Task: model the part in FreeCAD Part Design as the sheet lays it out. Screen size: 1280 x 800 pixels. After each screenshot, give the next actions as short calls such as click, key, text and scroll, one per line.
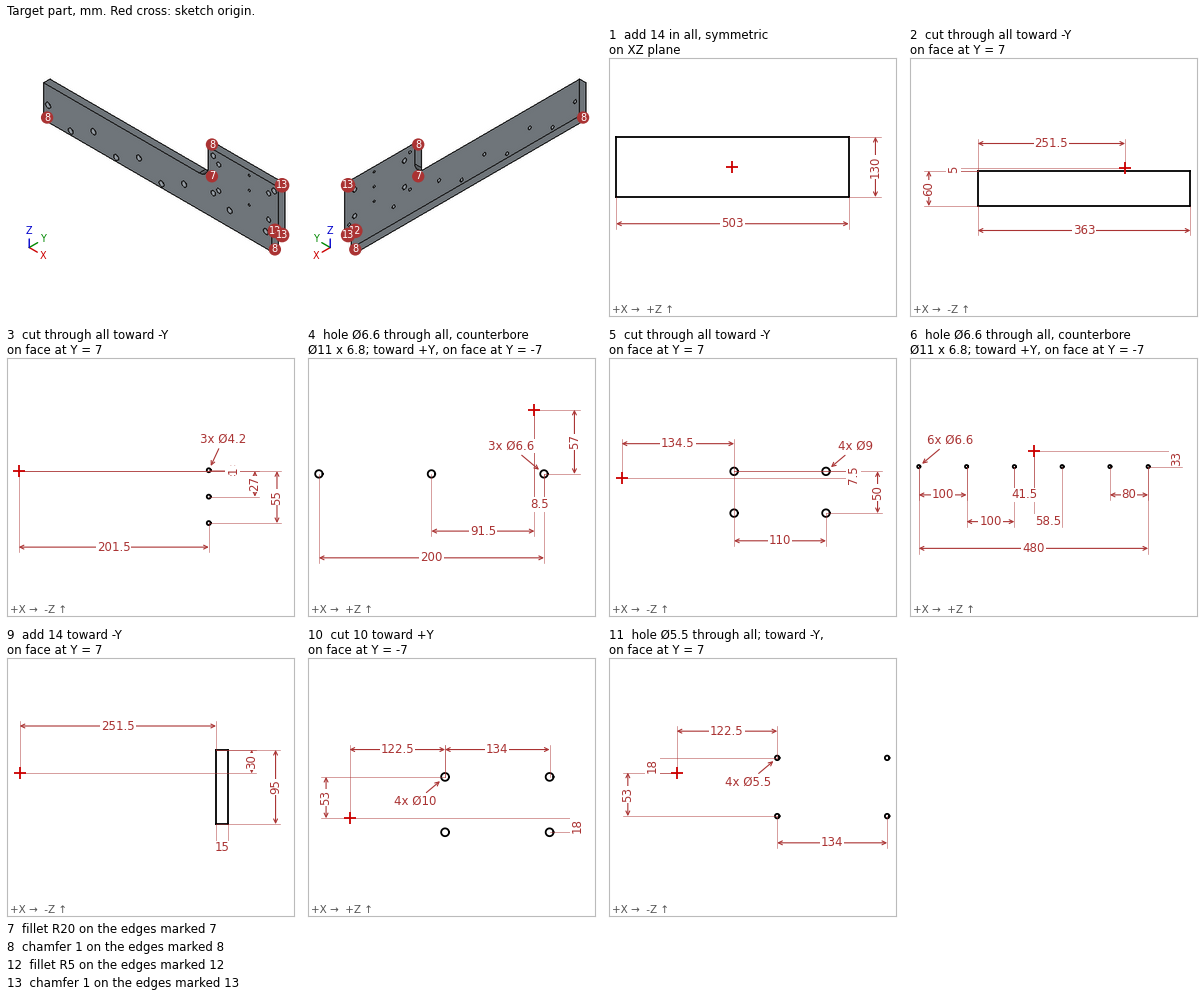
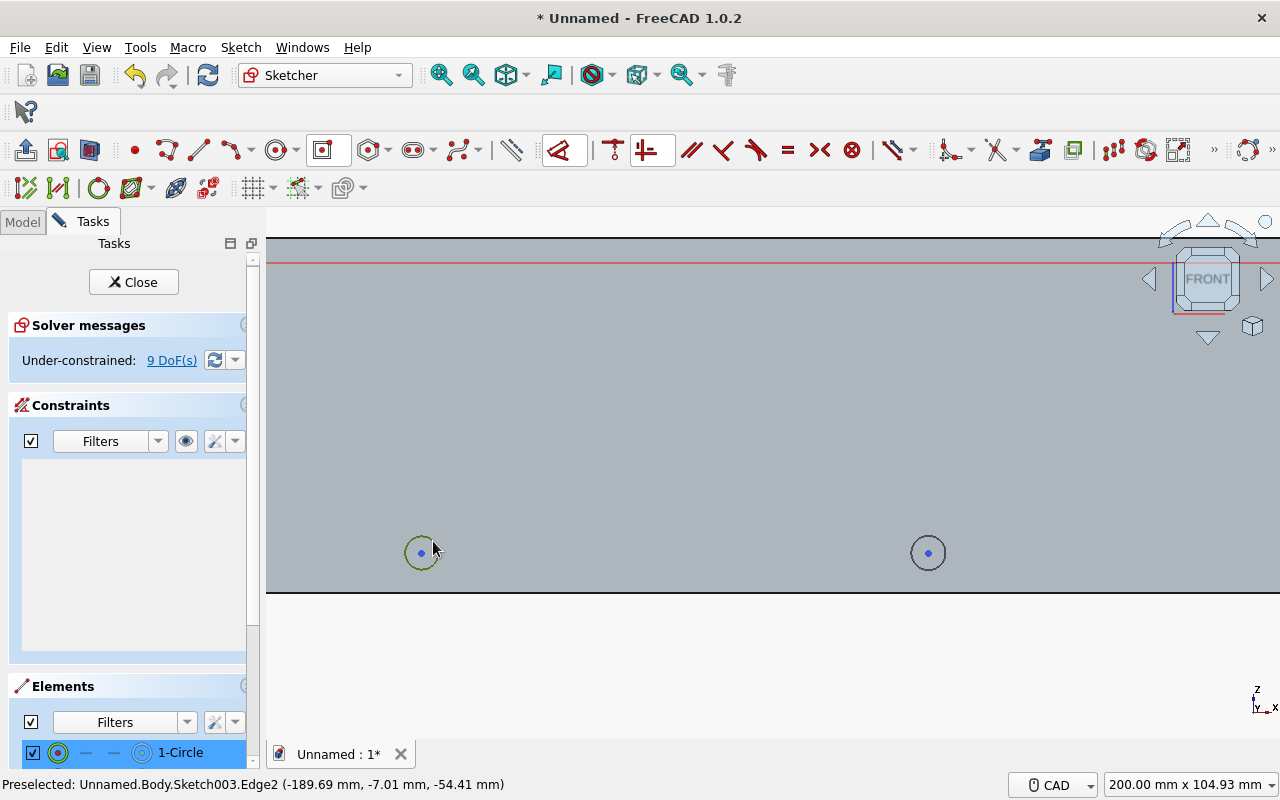
click(940, 541)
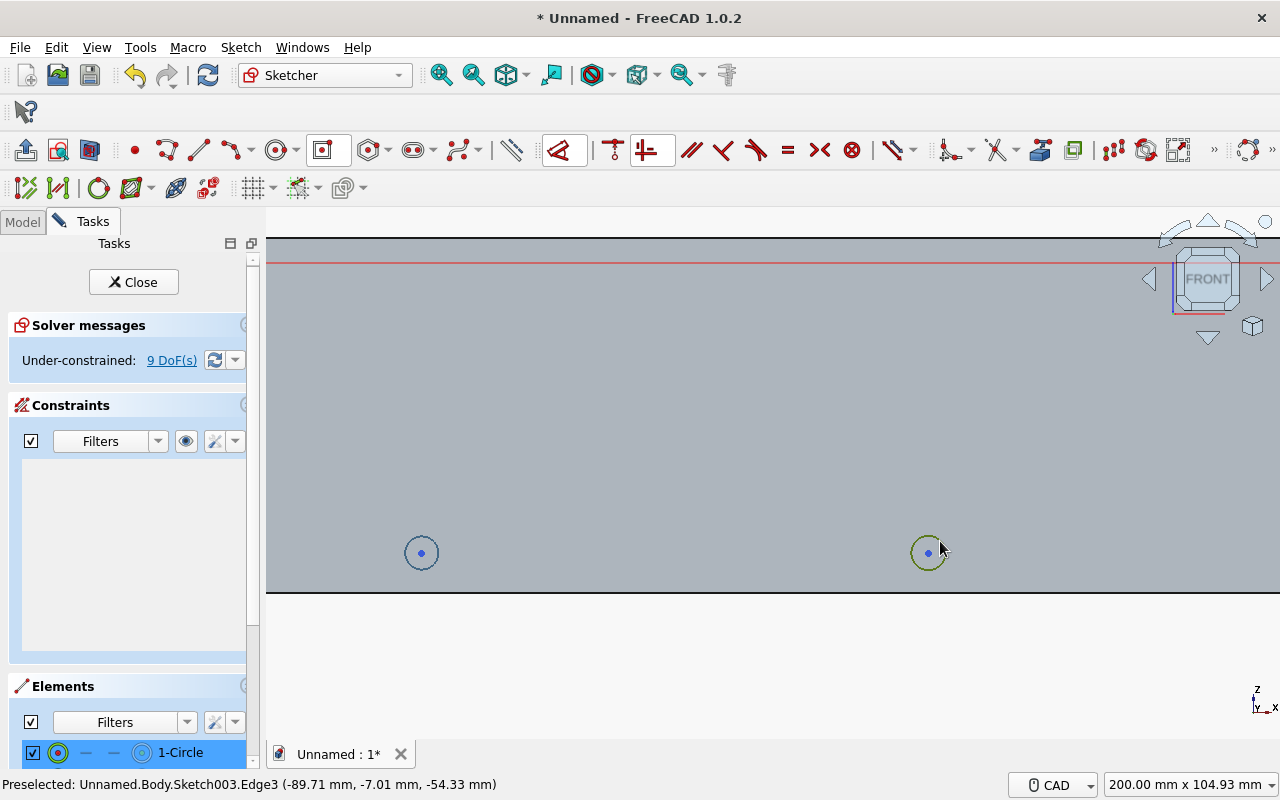
click(788, 150)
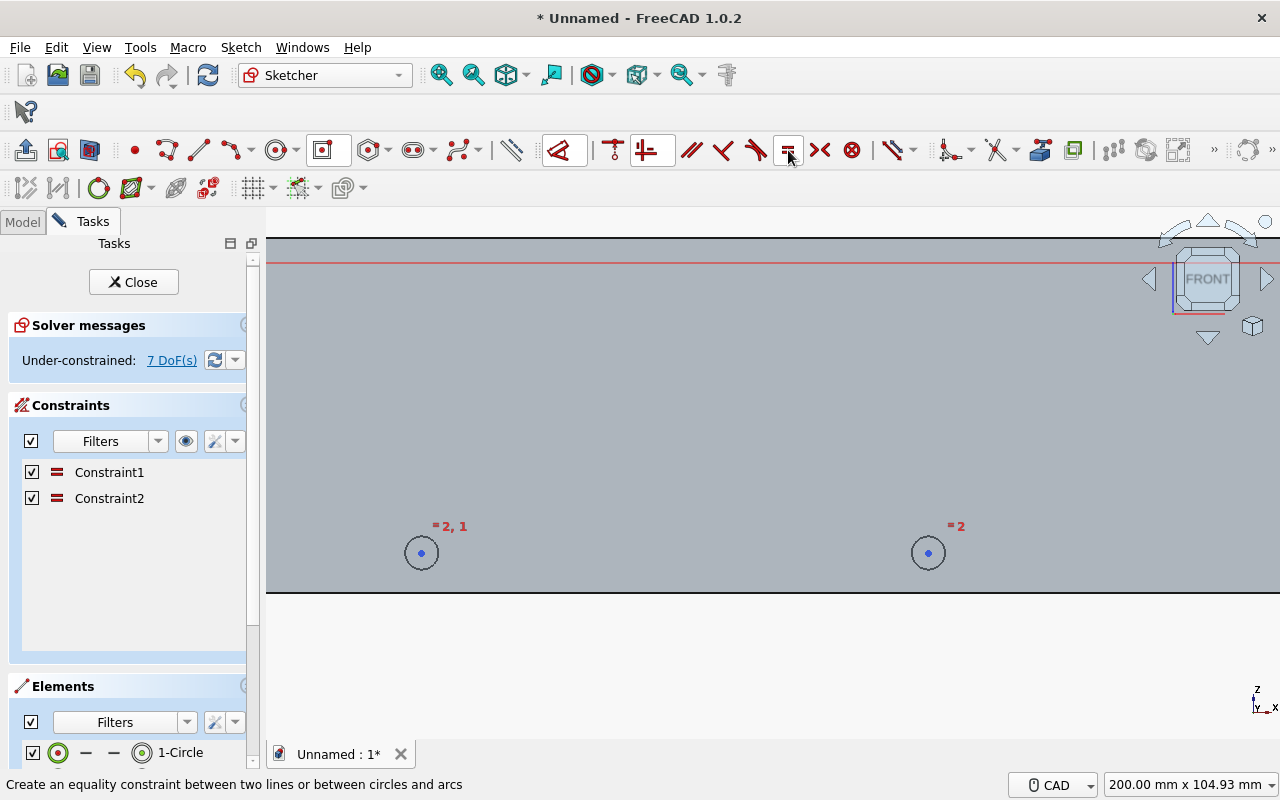
scroll(432, 542, down, 3)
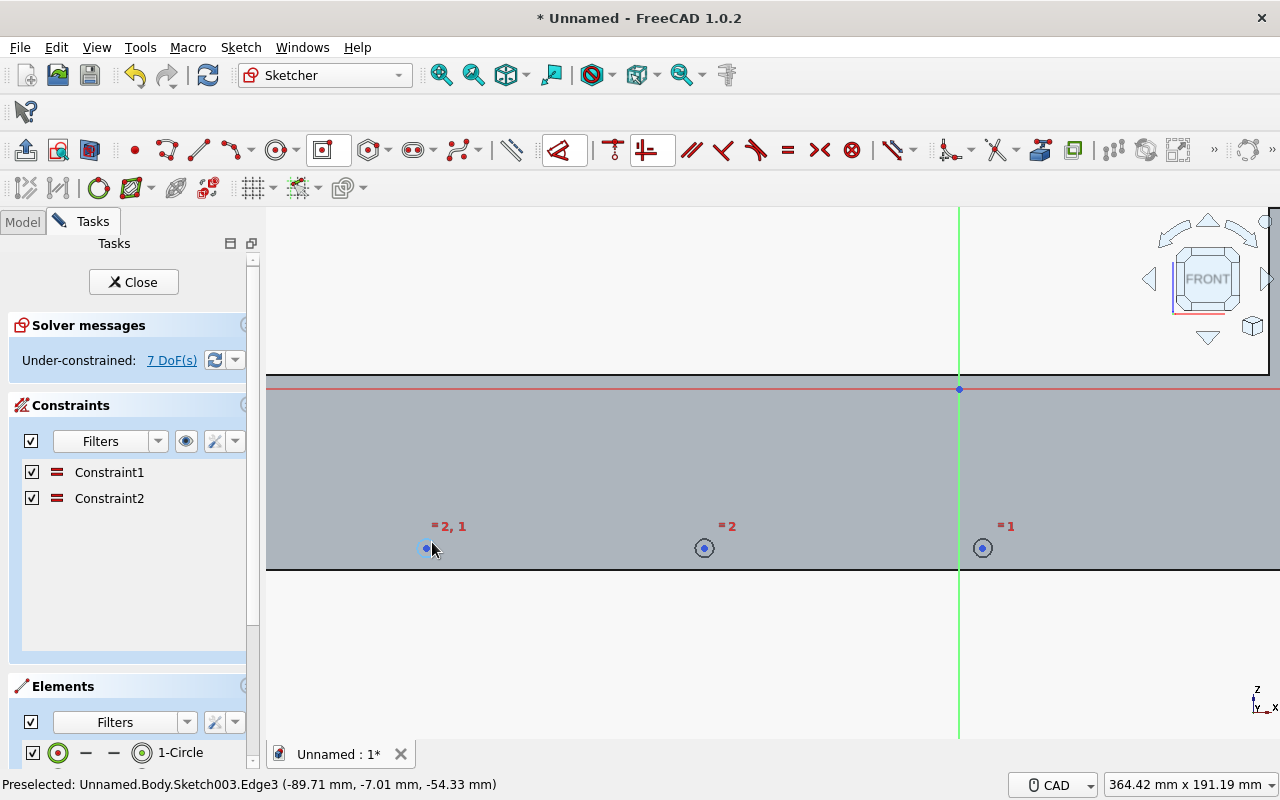
click(983, 548)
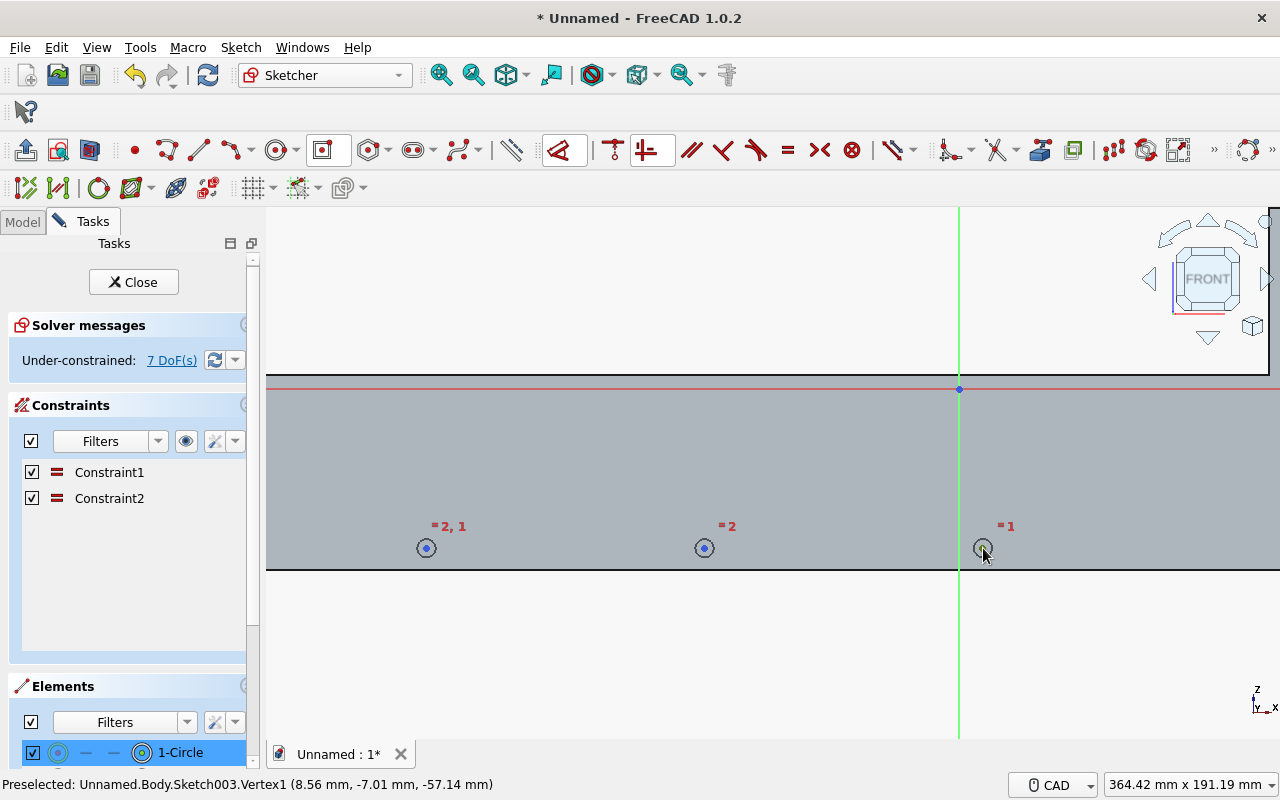
click(426, 548)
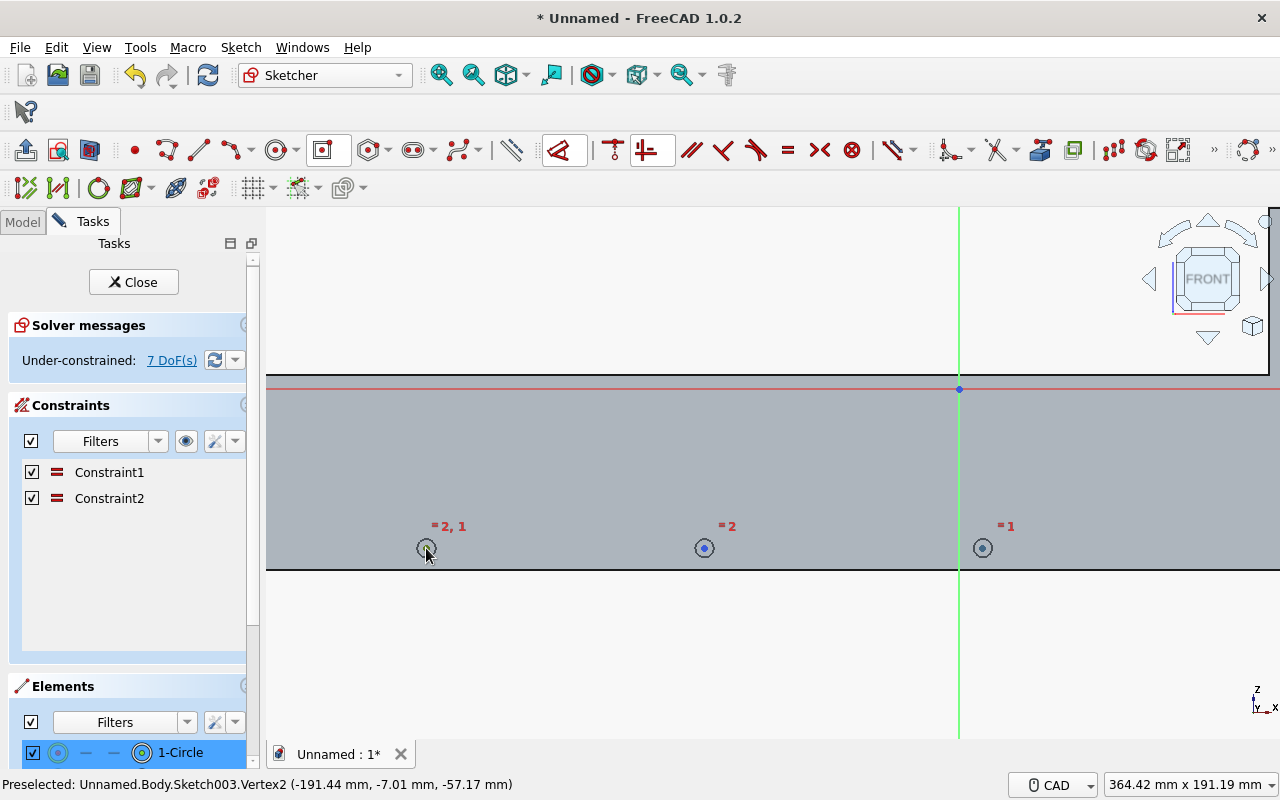
key(h)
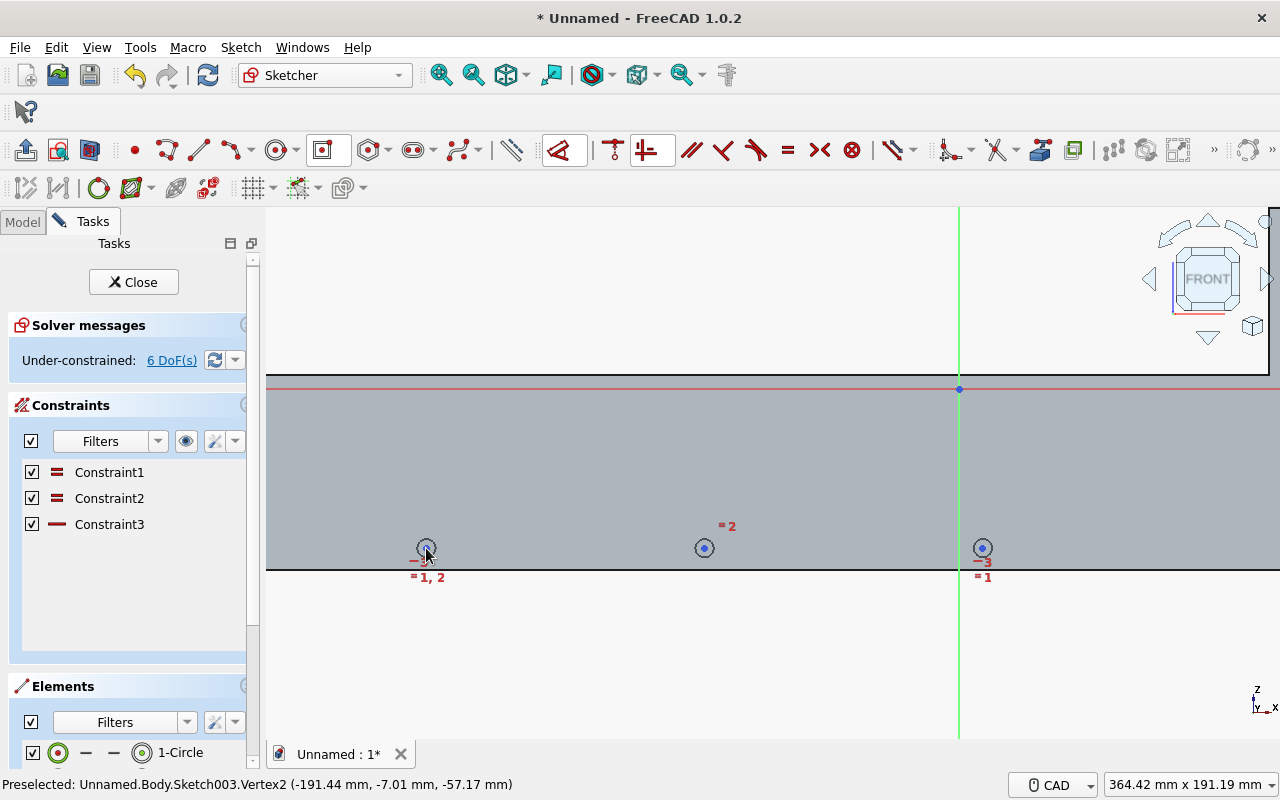
click(983, 548)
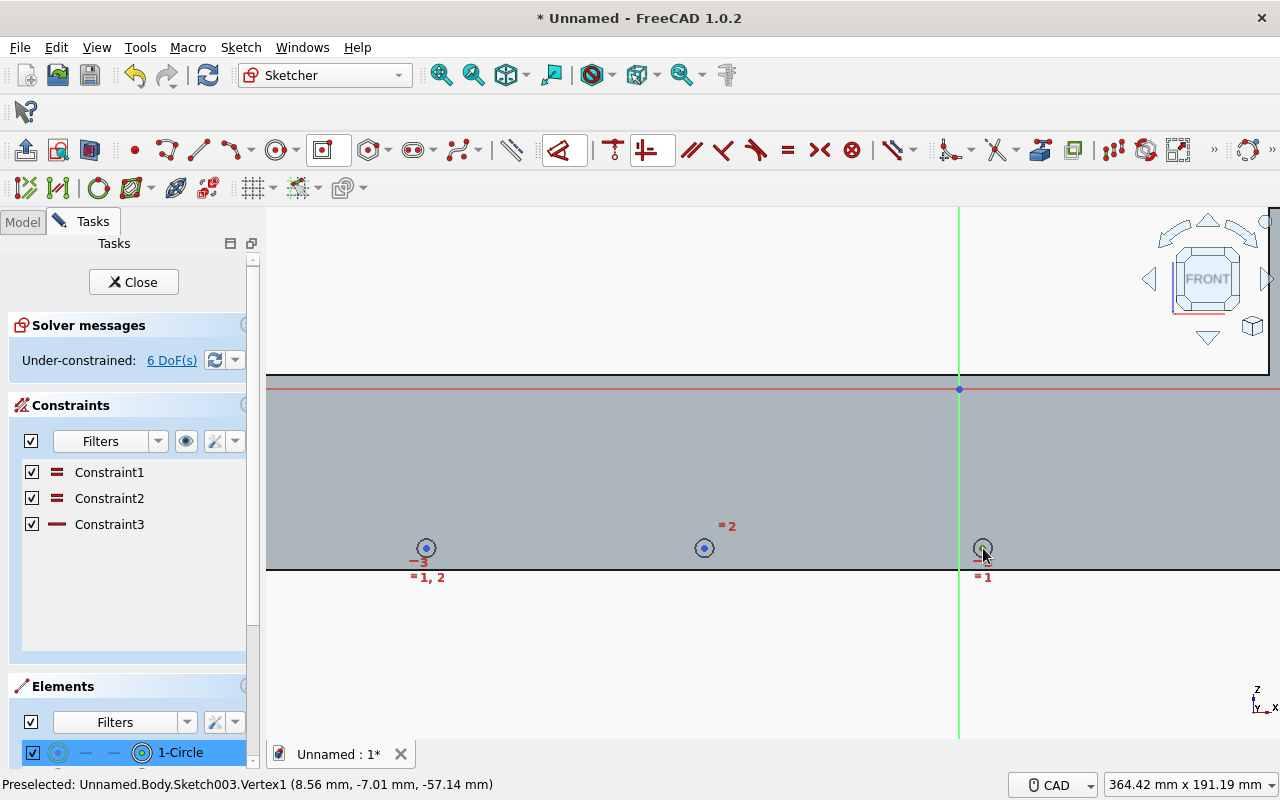
click(705, 548)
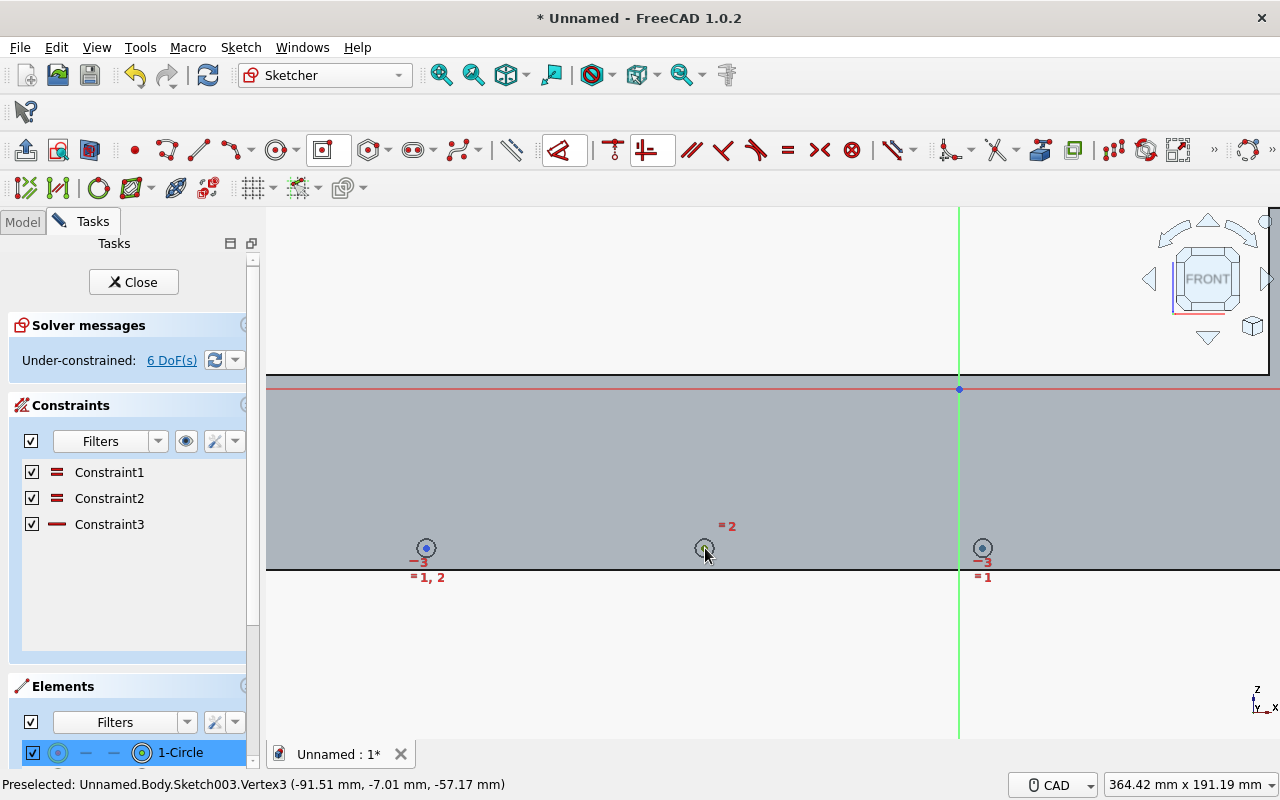
key(h)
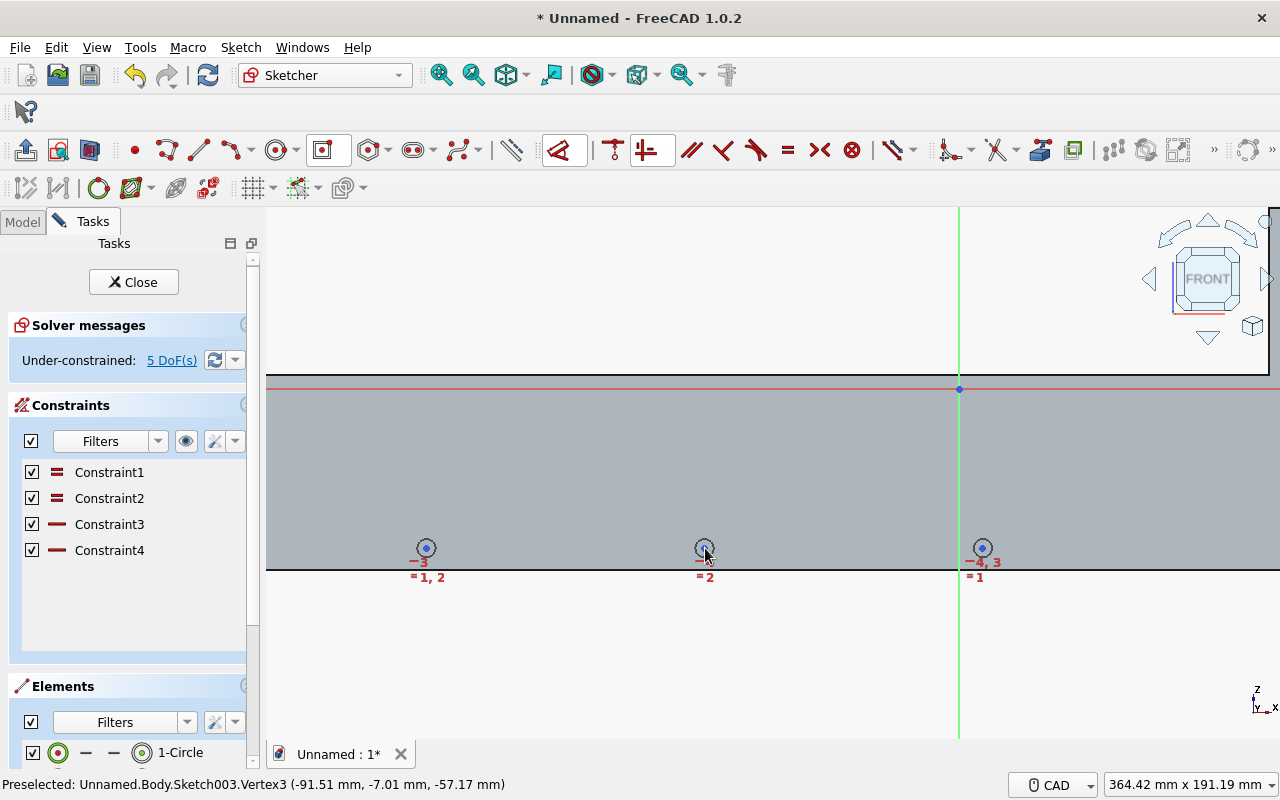
scroll(989, 542, up, 4)